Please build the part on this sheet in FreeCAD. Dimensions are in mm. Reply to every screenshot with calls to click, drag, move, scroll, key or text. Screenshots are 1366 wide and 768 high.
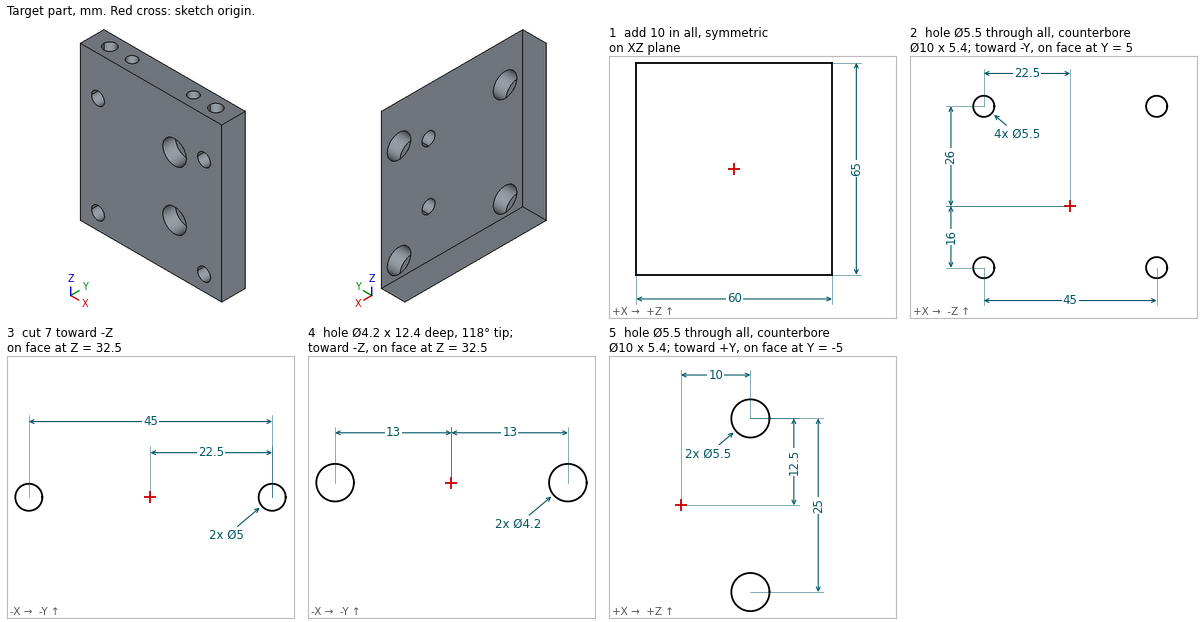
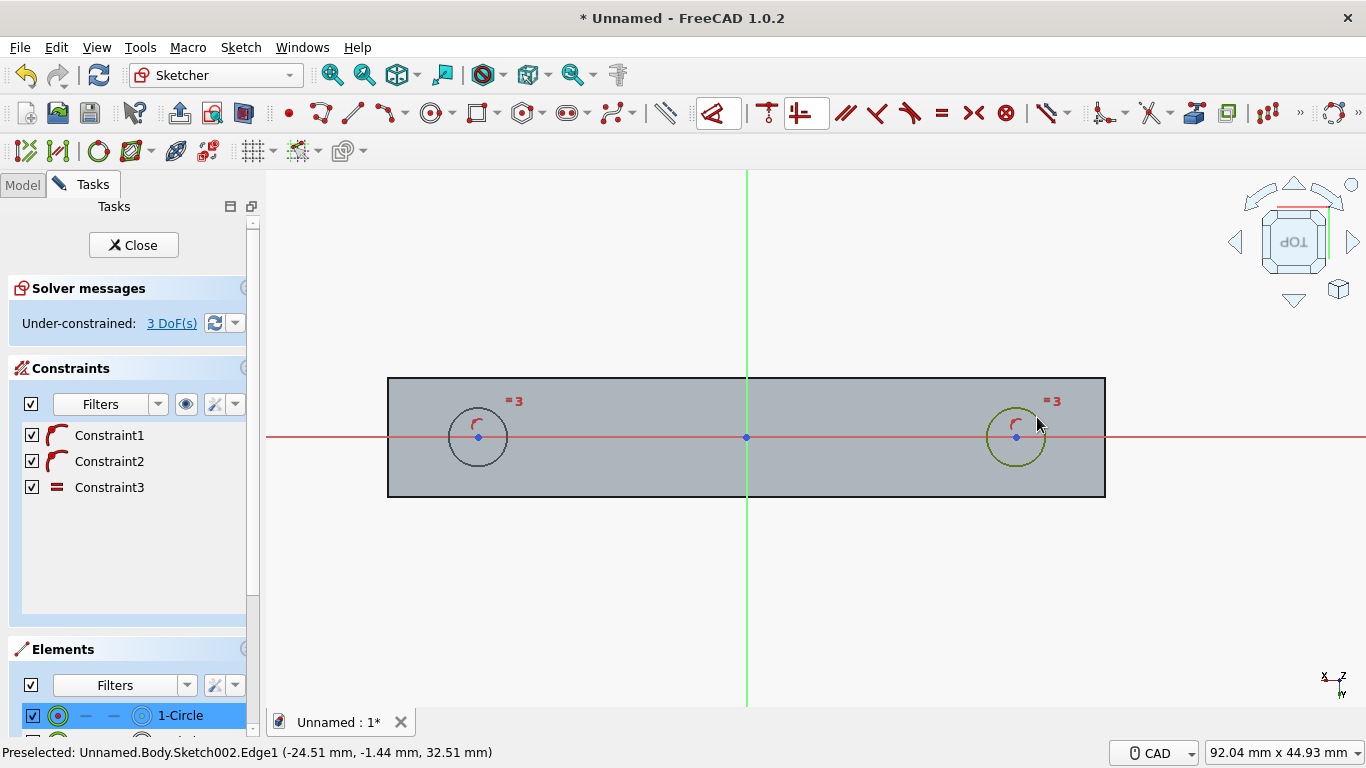
key(k)
key(o)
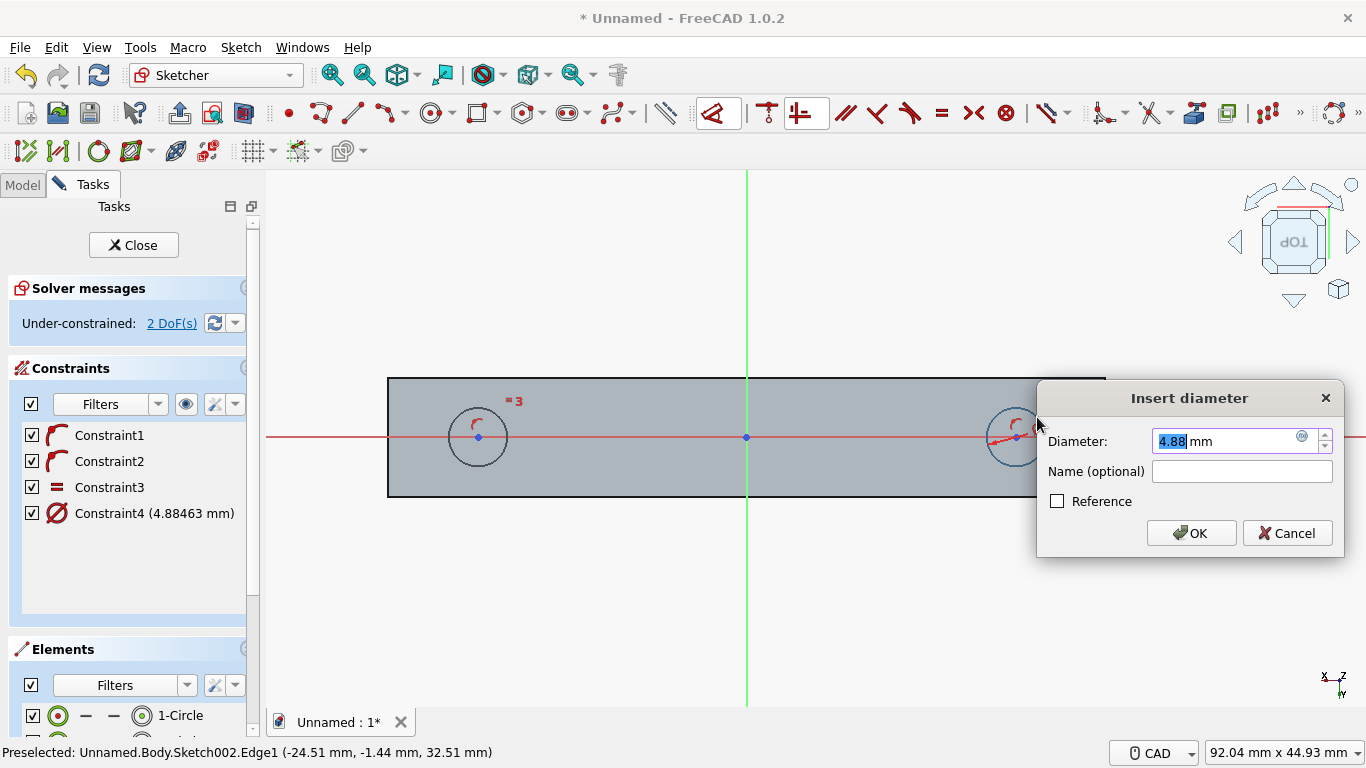
text(5)
key(Return)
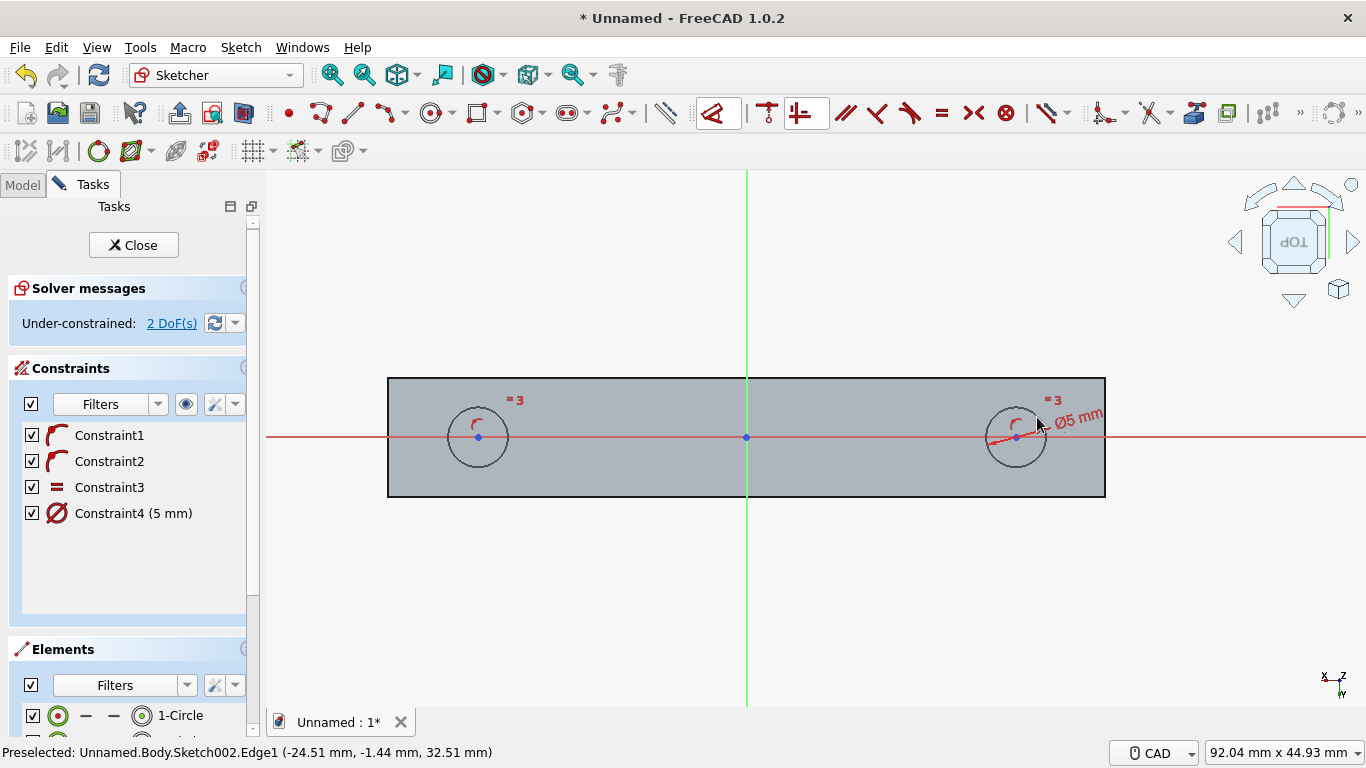
click(1016, 437)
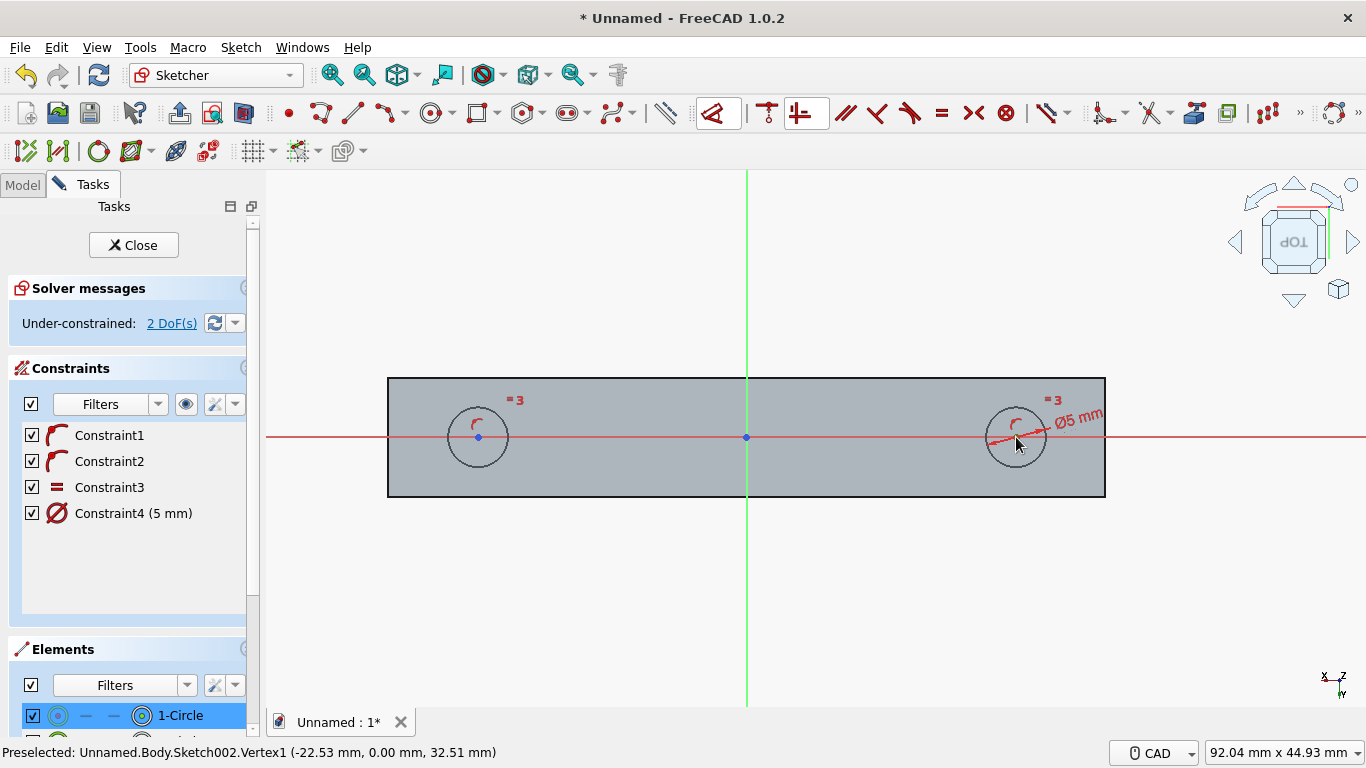
click(478, 437)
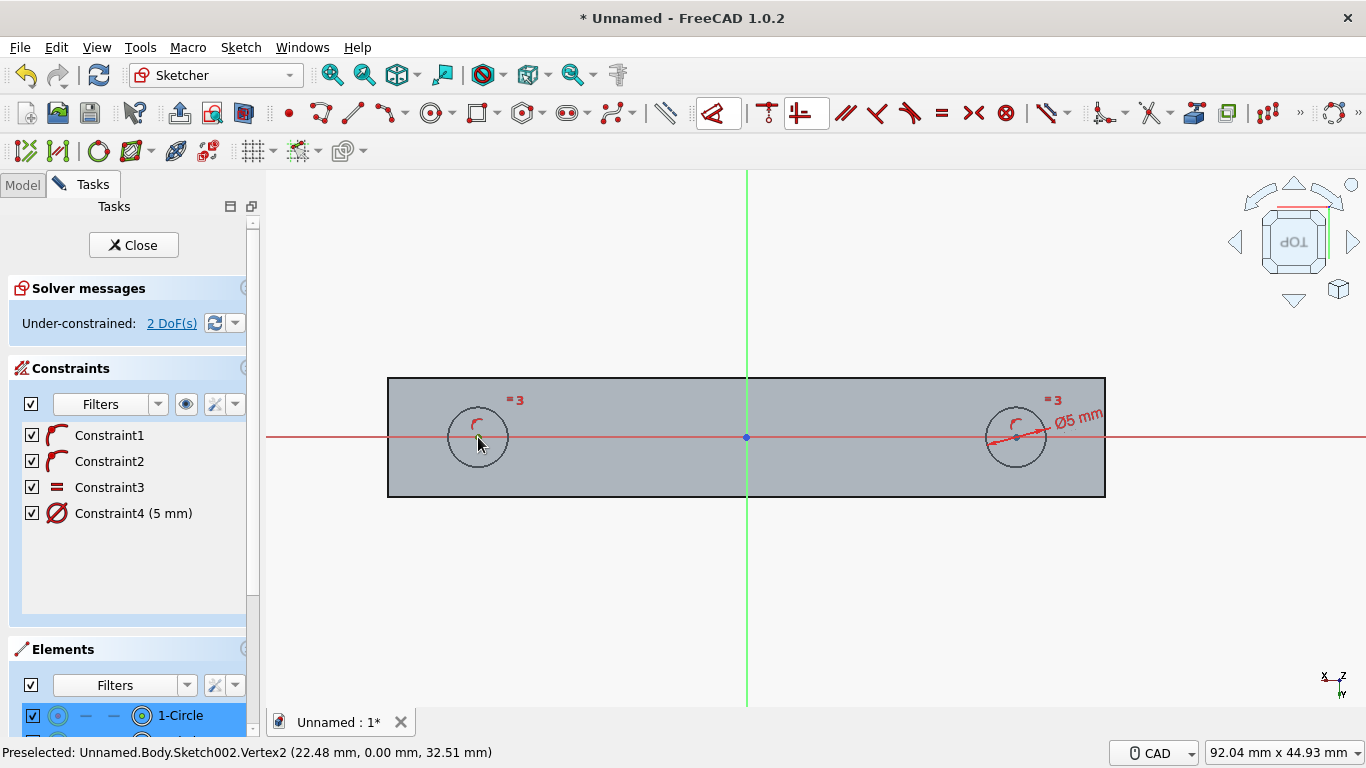
key(l)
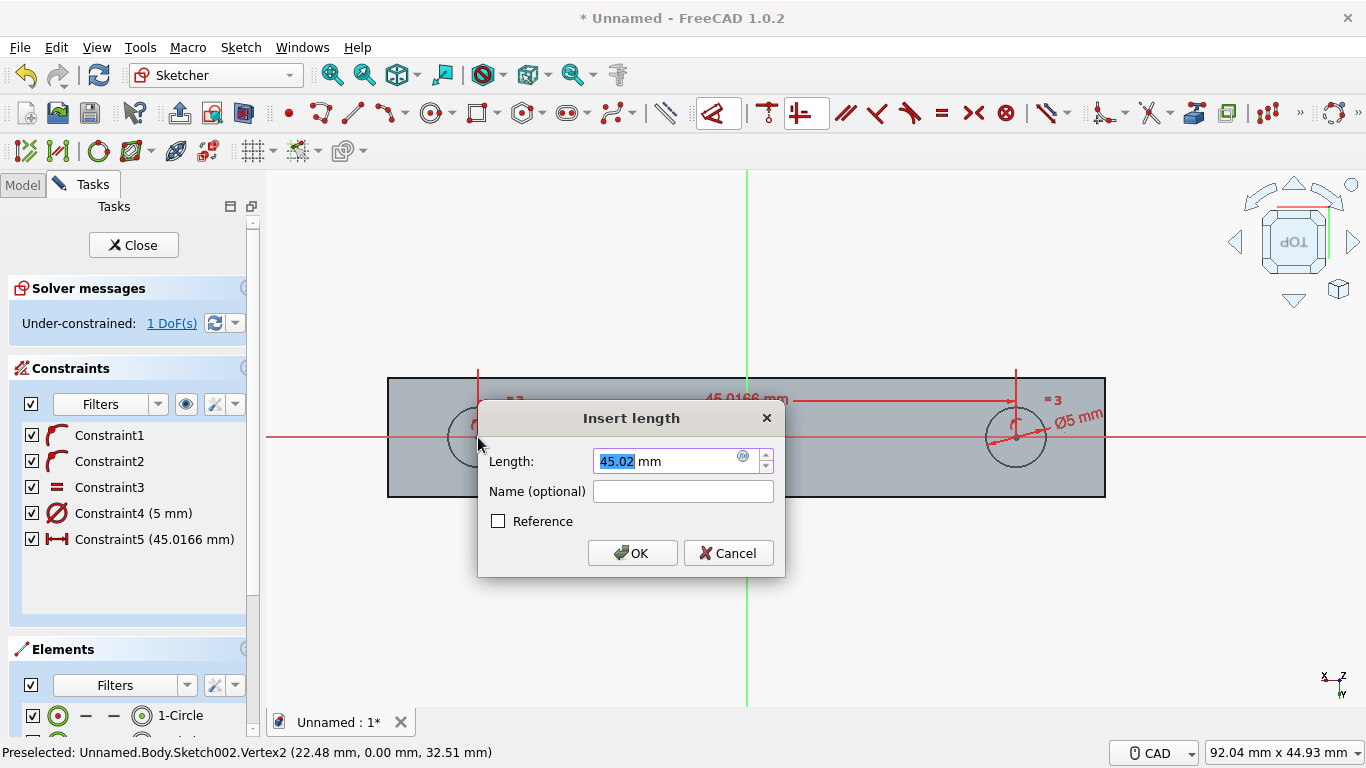
text(45)
key(Return)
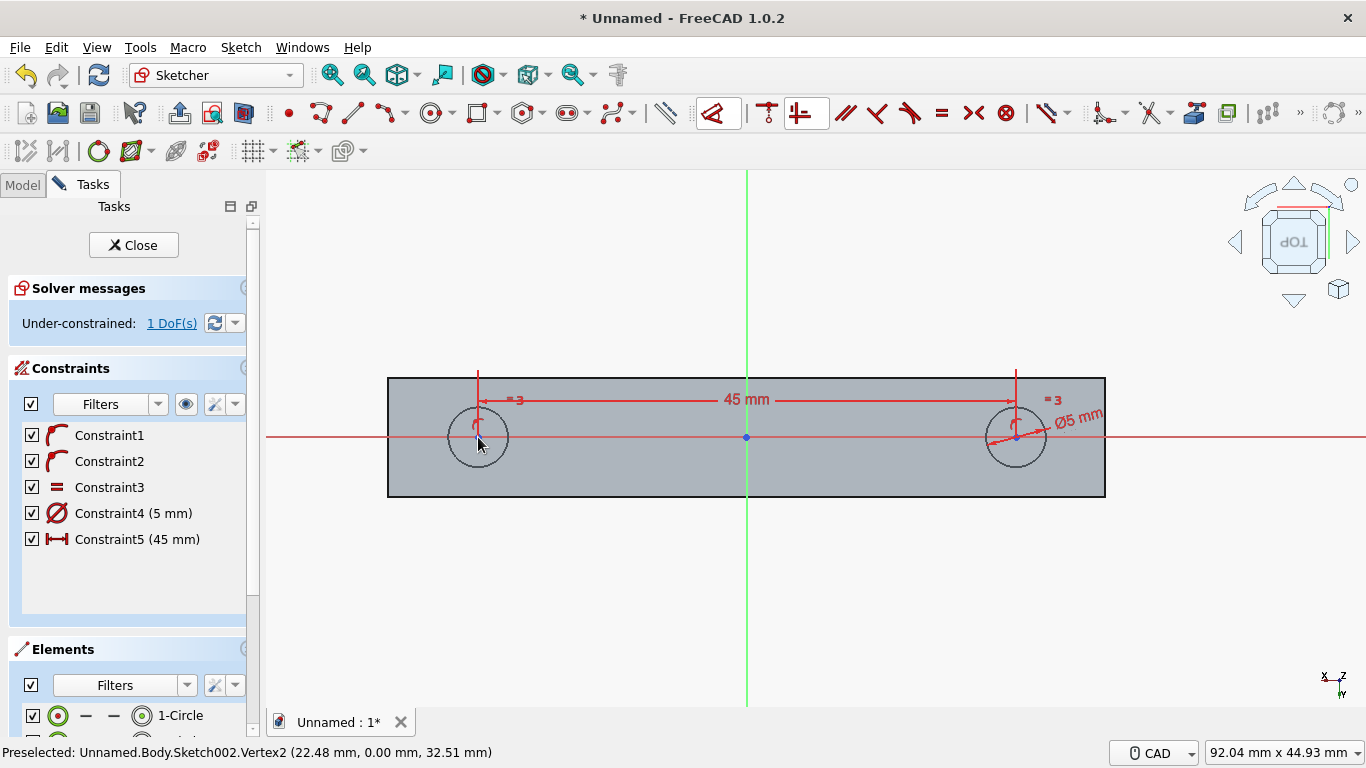
click(1016, 437)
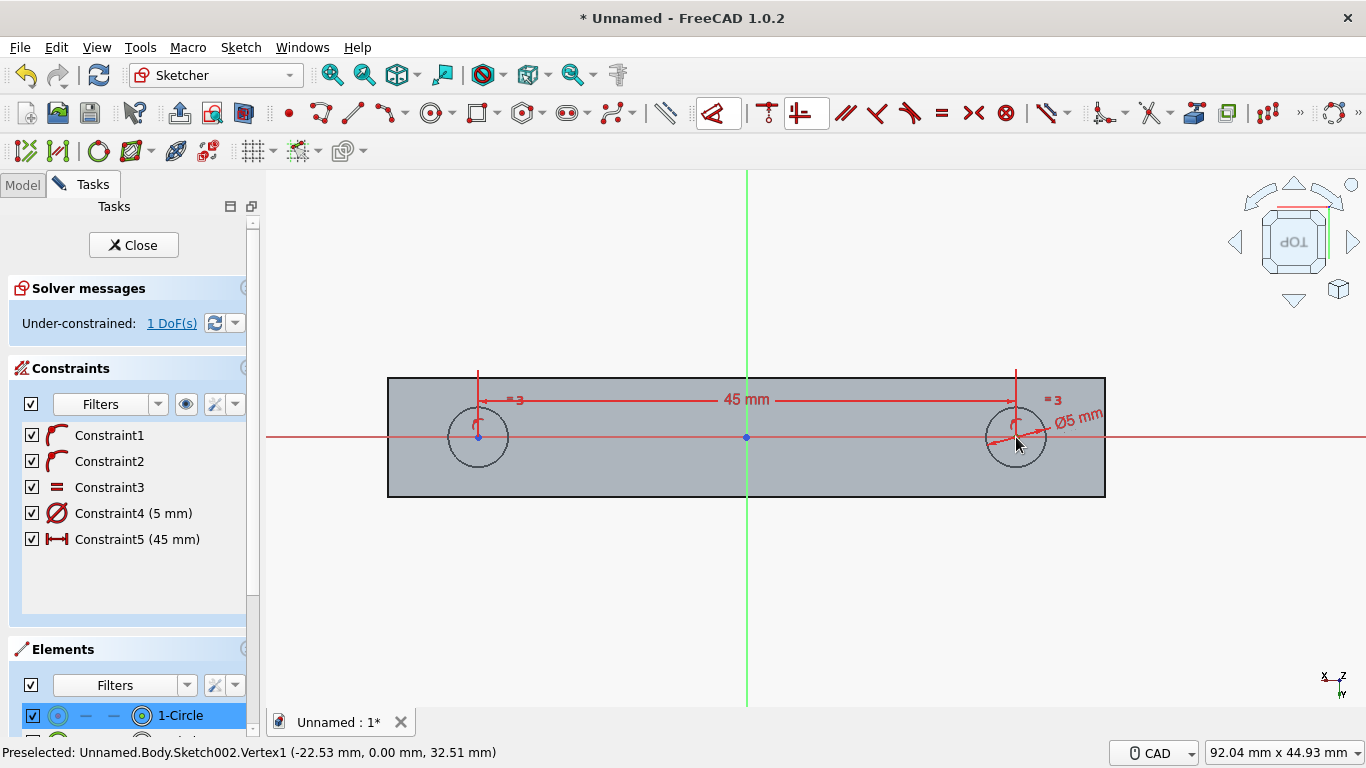
key(l)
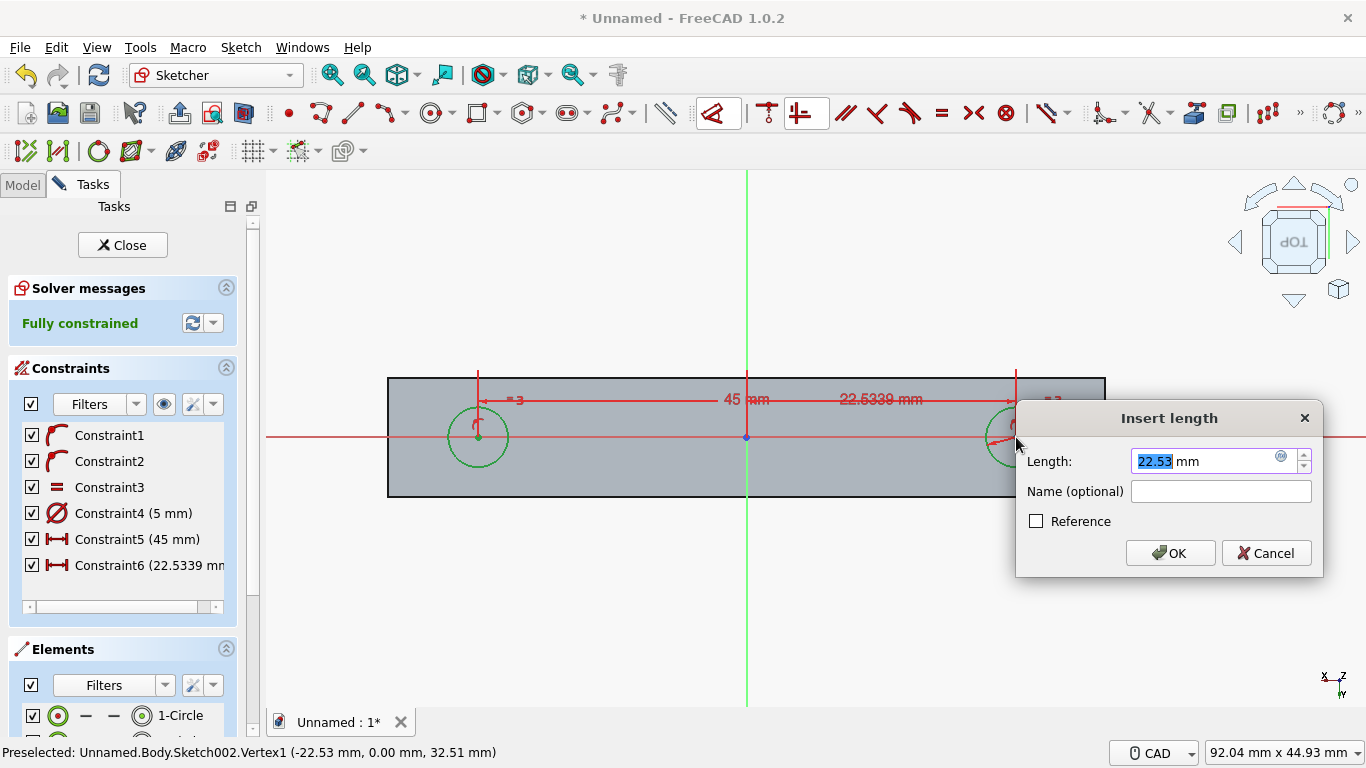
text(22.5)
key(Return)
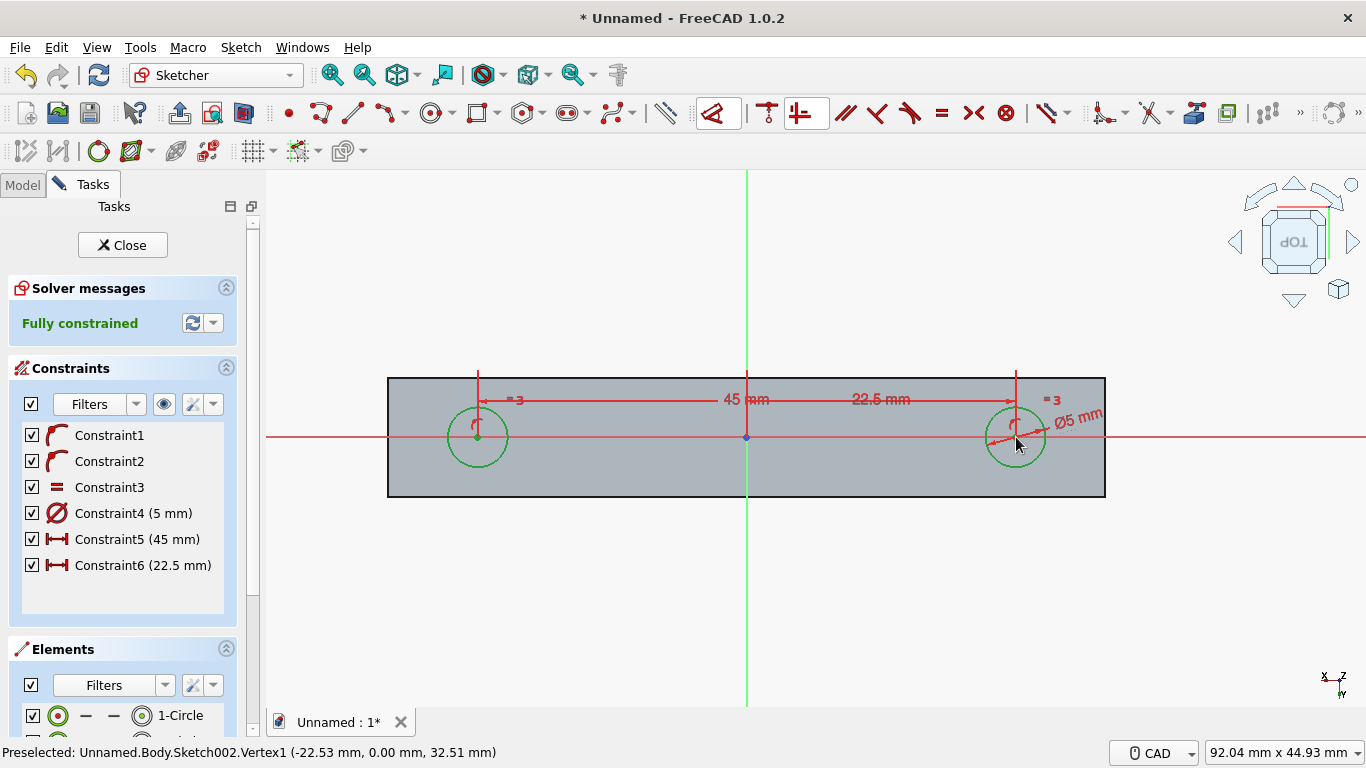
click(123, 245)